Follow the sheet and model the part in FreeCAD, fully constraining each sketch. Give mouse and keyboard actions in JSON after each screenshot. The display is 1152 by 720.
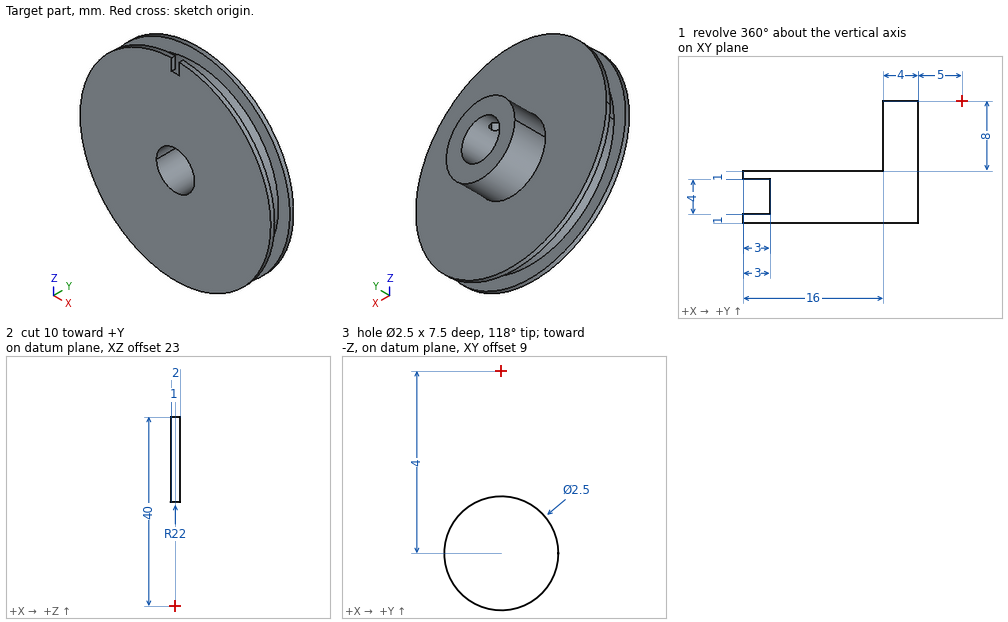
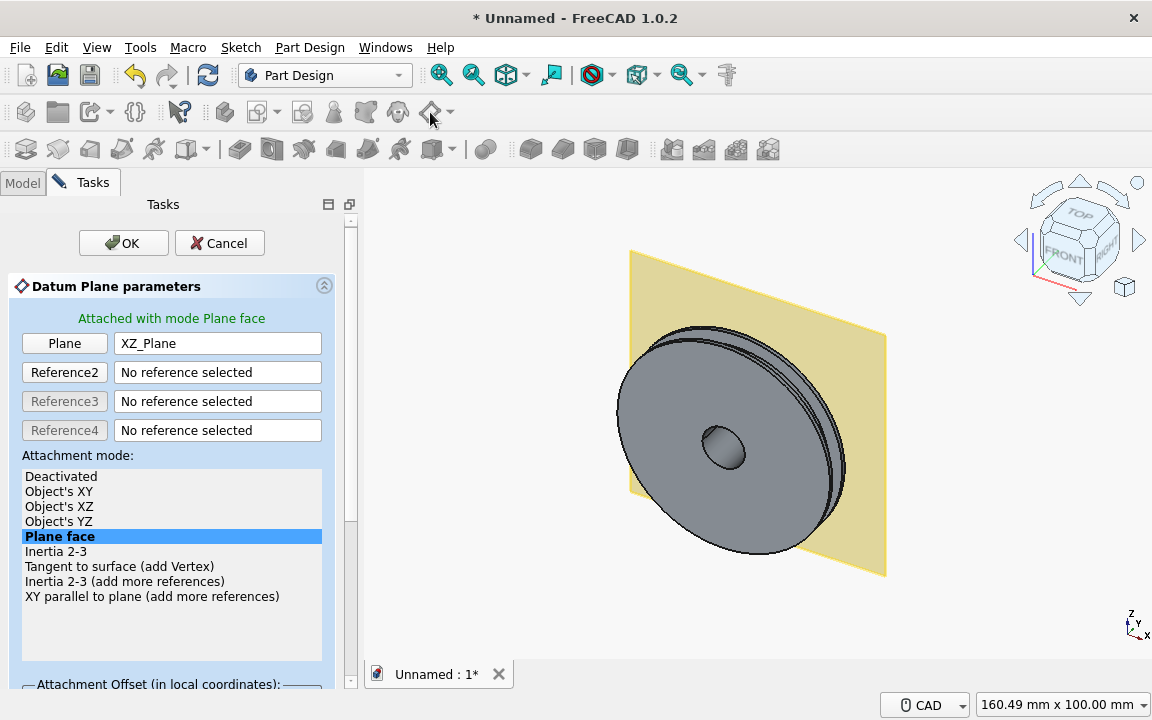
{"action": "scroll", "coordinate": [351, 451], "scroll_direction": "down", "scroll_amount": 3}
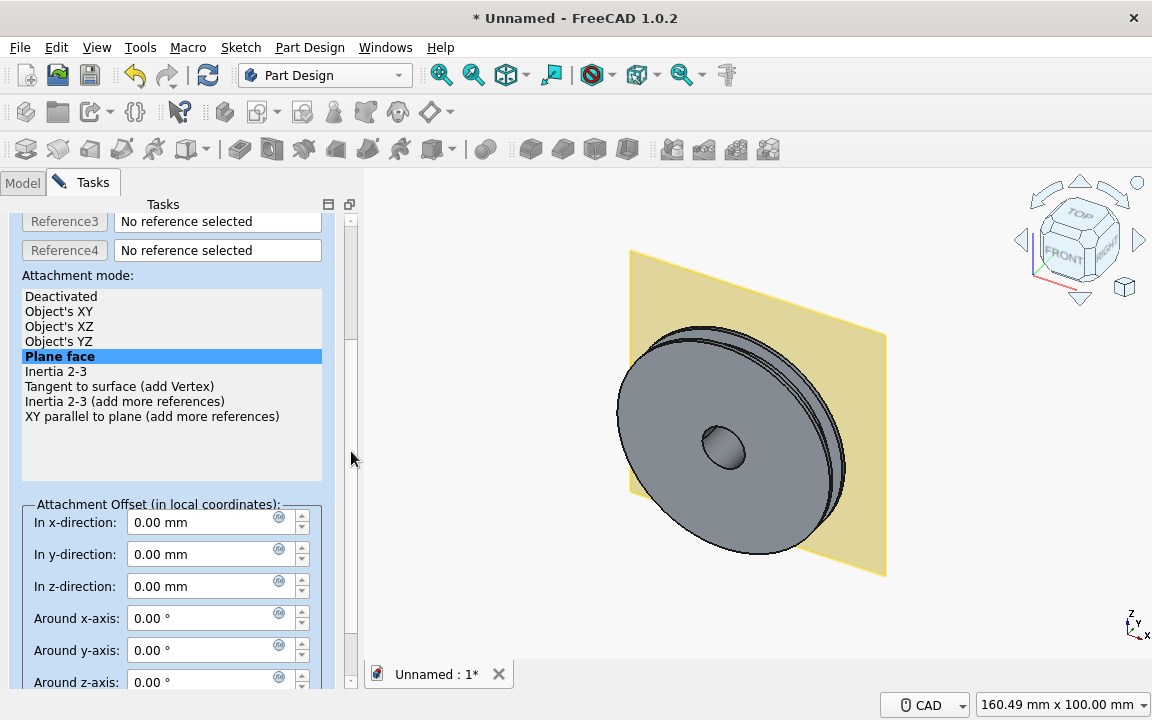
{"action": "triple_click", "coordinate": [210, 586]}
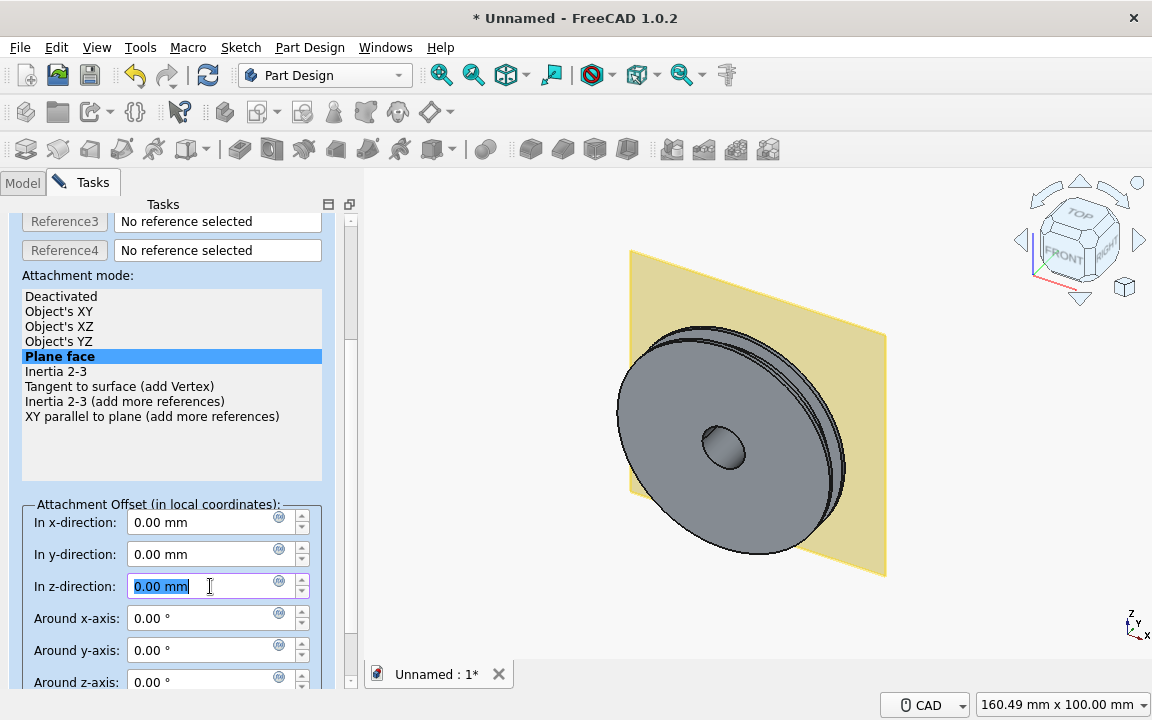
{"action": "type", "text": "23"}
{"action": "key", "text": "Tab"}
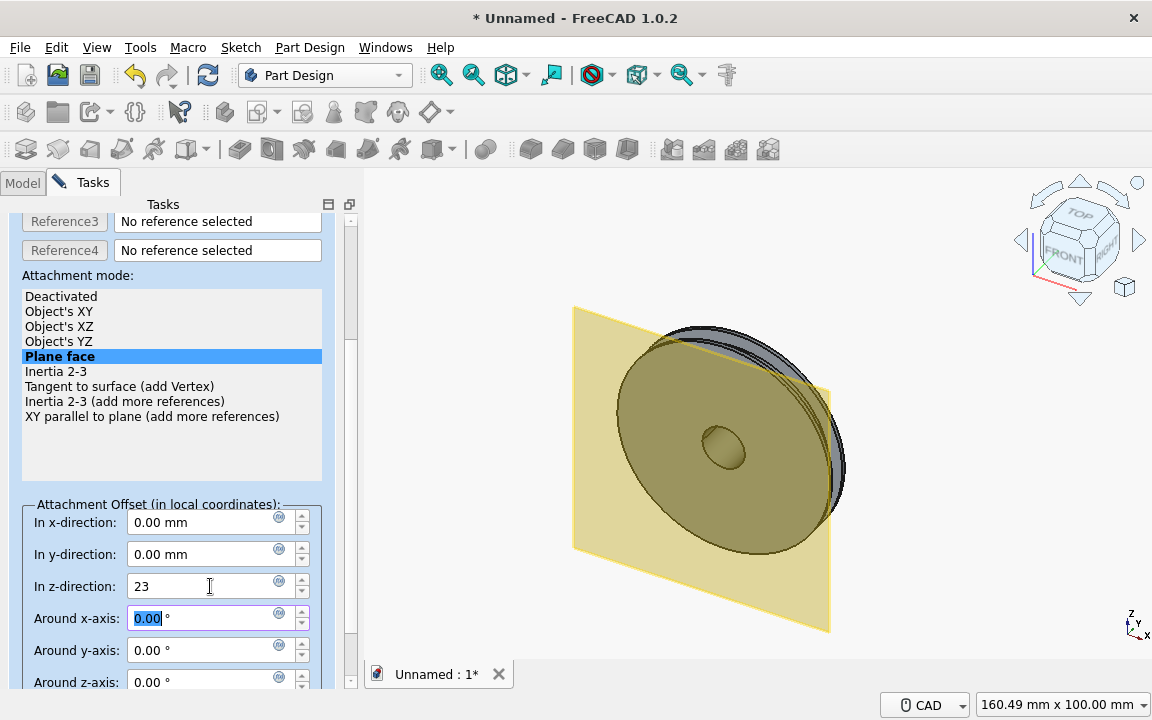
{"action": "scroll", "coordinate": [351, 451], "scroll_direction": "up", "scroll_amount": 4}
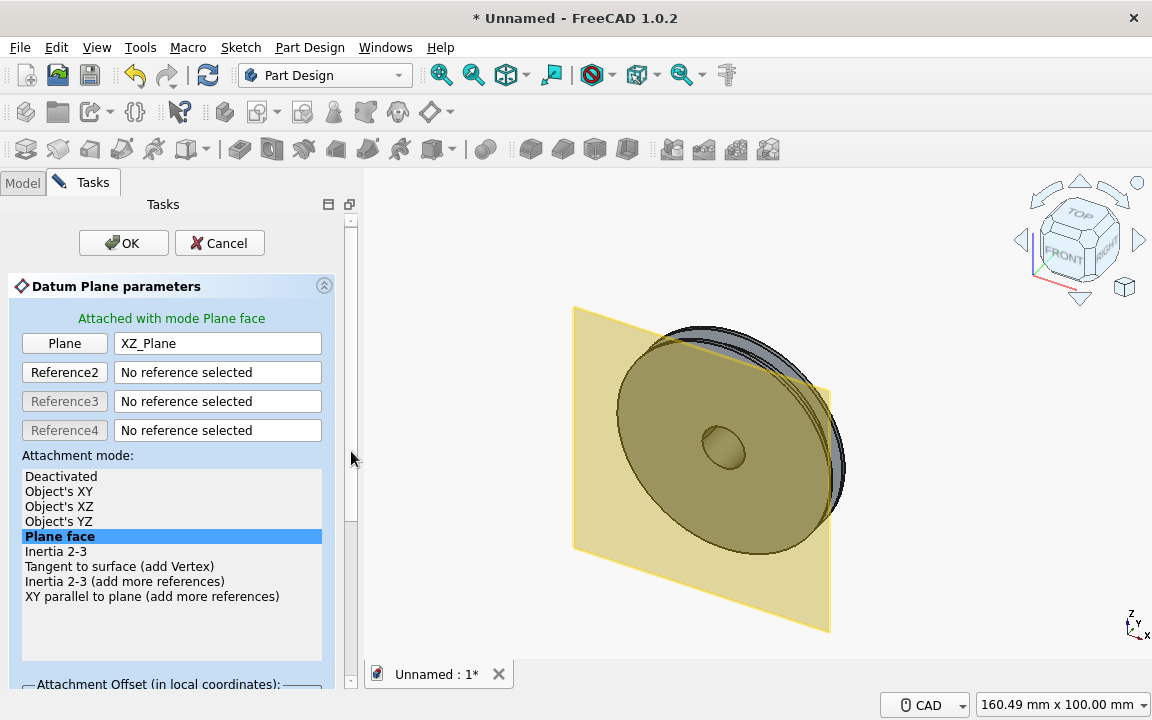
{"action": "left_click", "coordinate": [124, 243]}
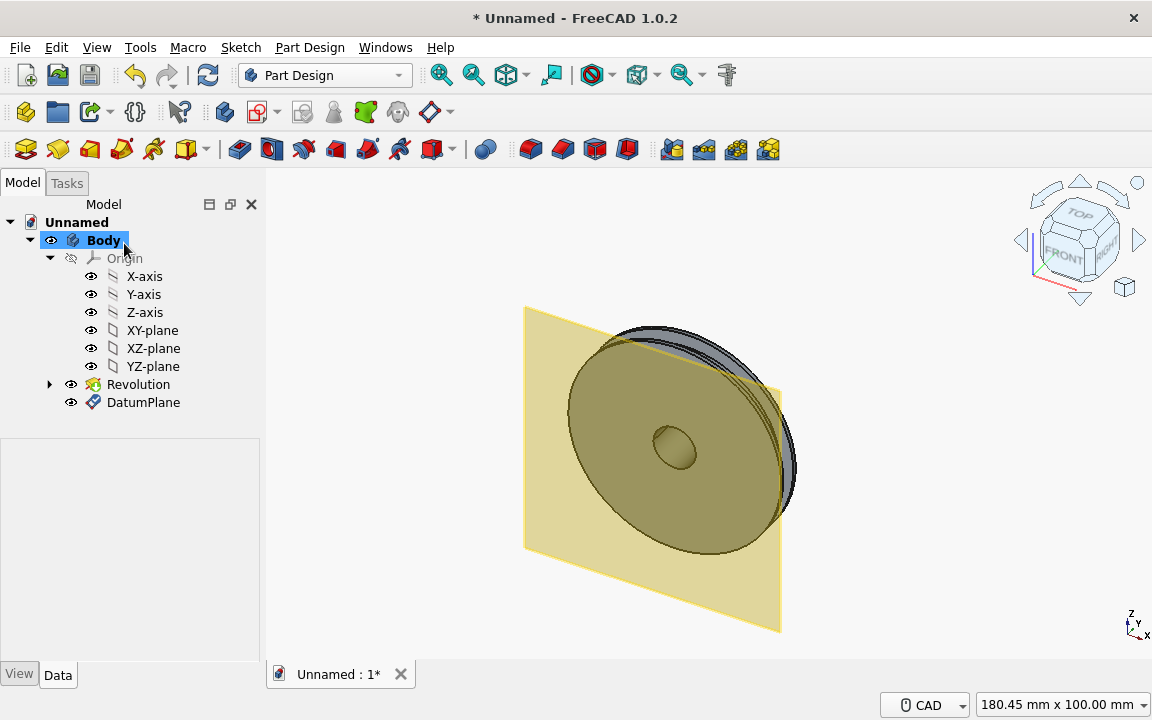
{"action": "left_click", "coordinate": [116, 402]}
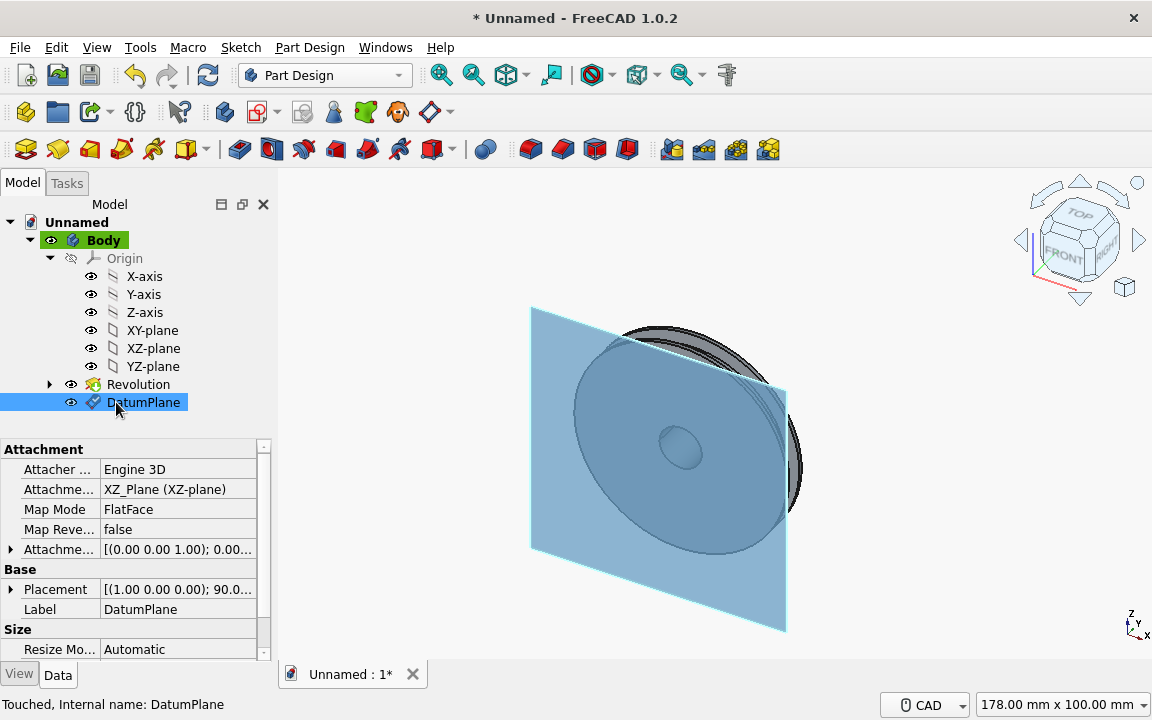
{"action": "left_click", "coordinate": [258, 112]}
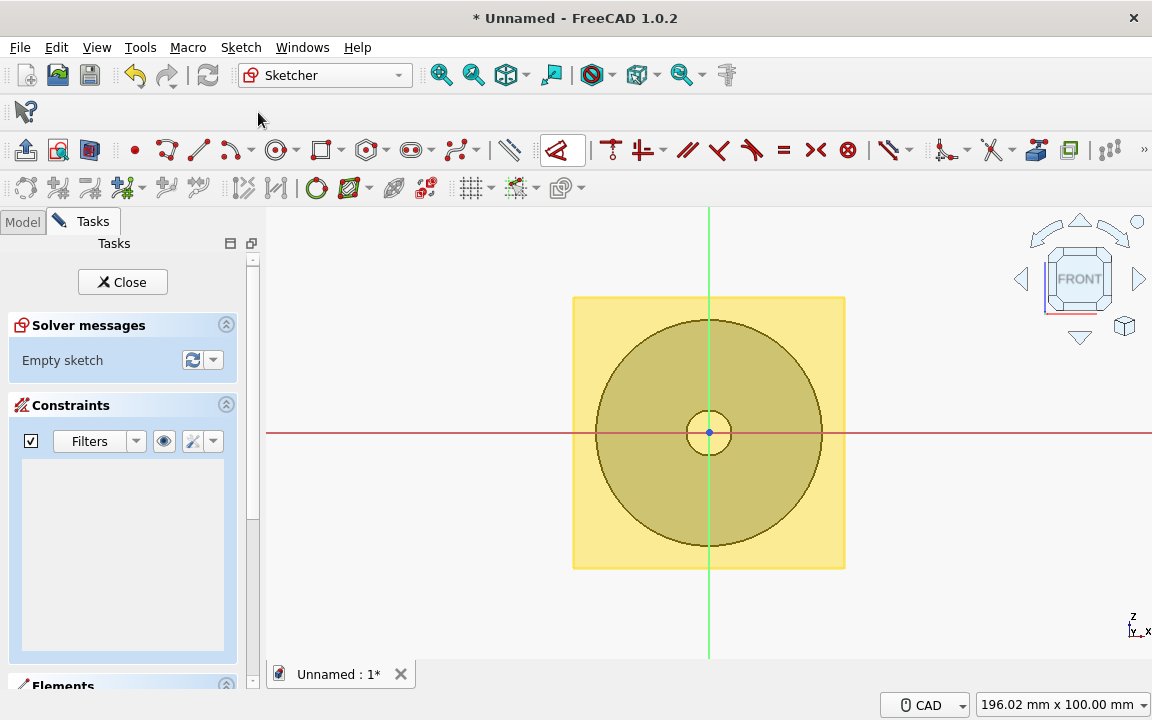
{"action": "scroll", "coordinate": [848, 235], "scroll_direction": "up", "scroll_amount": 2}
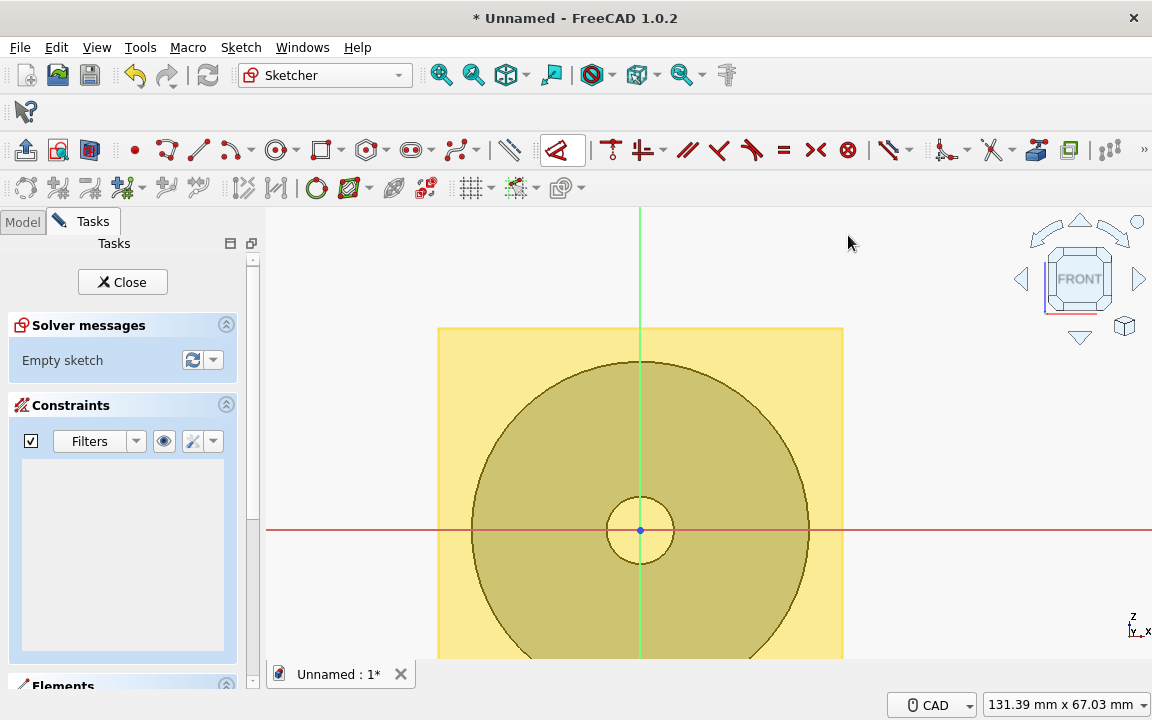
{"action": "key", "text": "g m"}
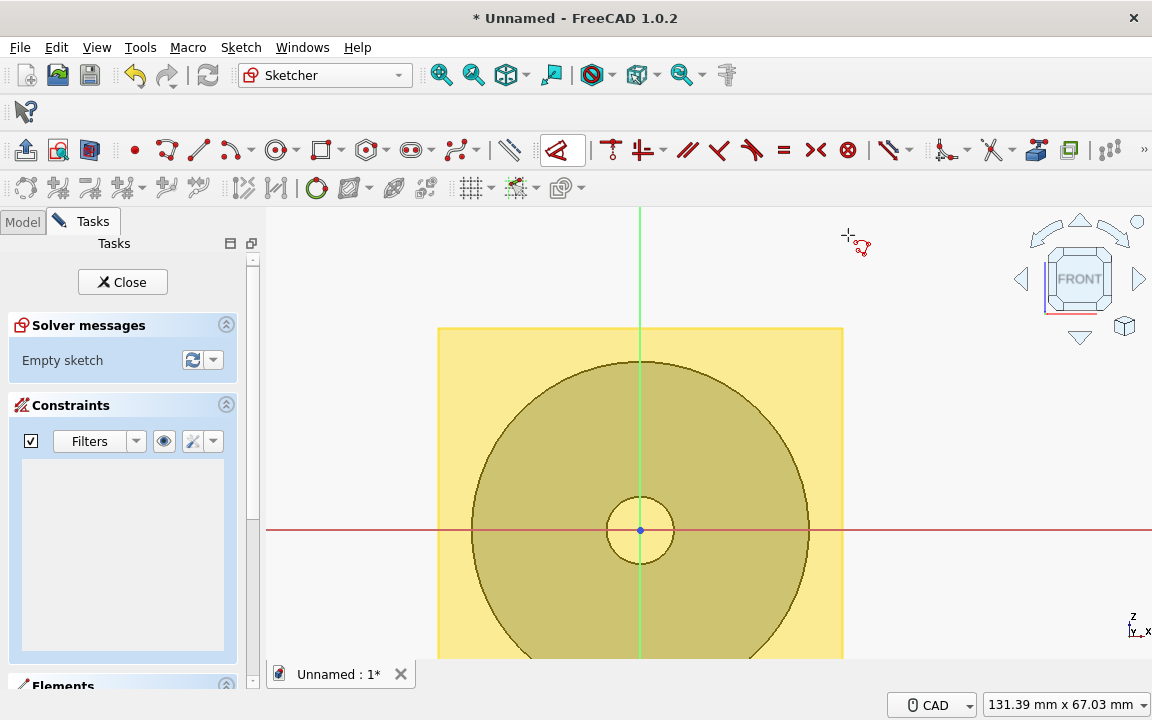
{"action": "scroll", "coordinate": [634, 382], "scroll_direction": "up", "scroll_amount": 5}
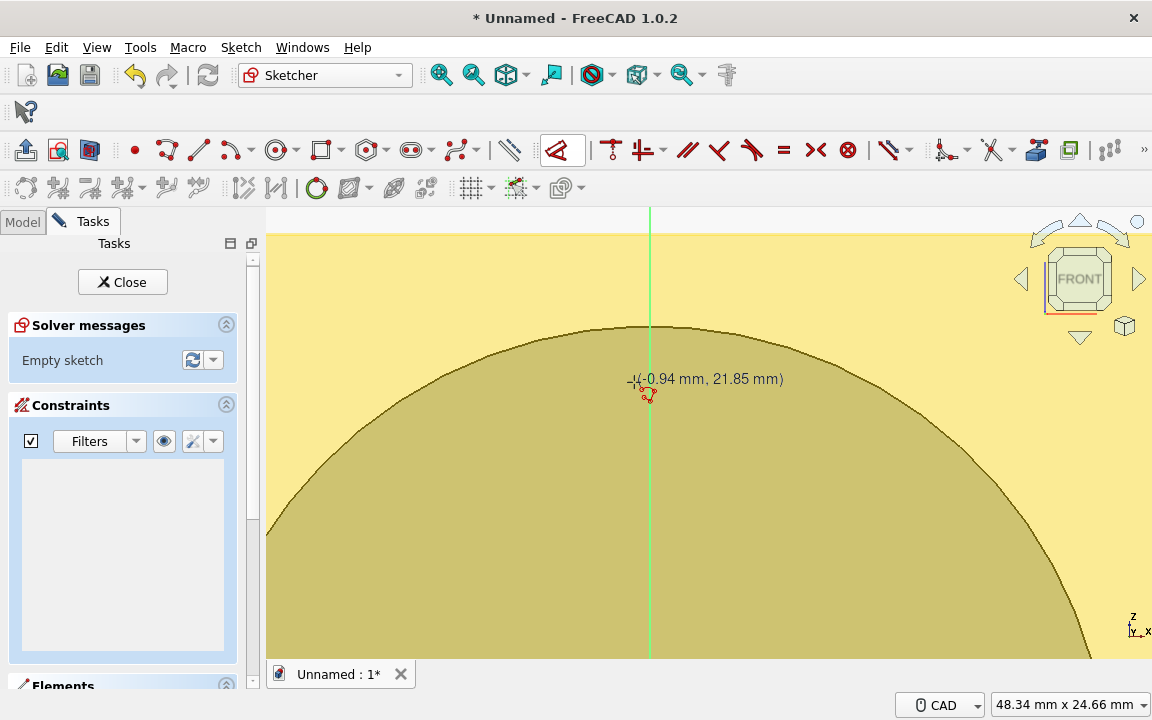
{"action": "left_click", "coordinate": [632, 382]}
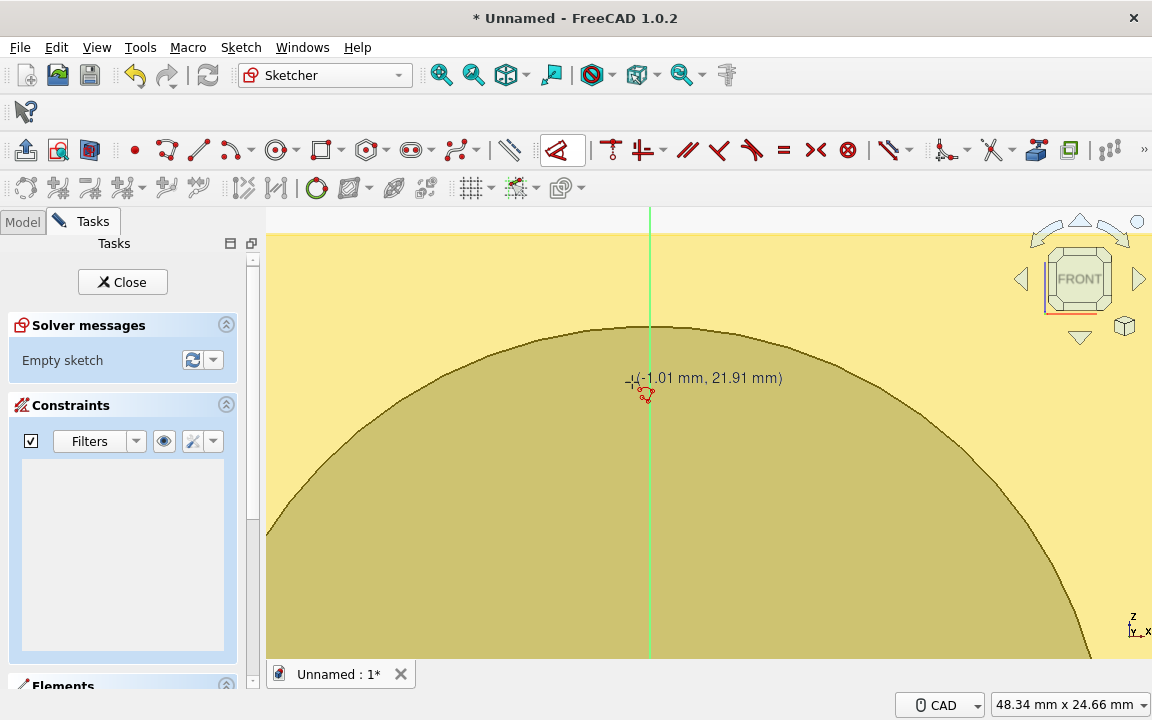
{"action": "scroll", "coordinate": [635, 442], "scroll_direction": "down", "scroll_amount": 5}